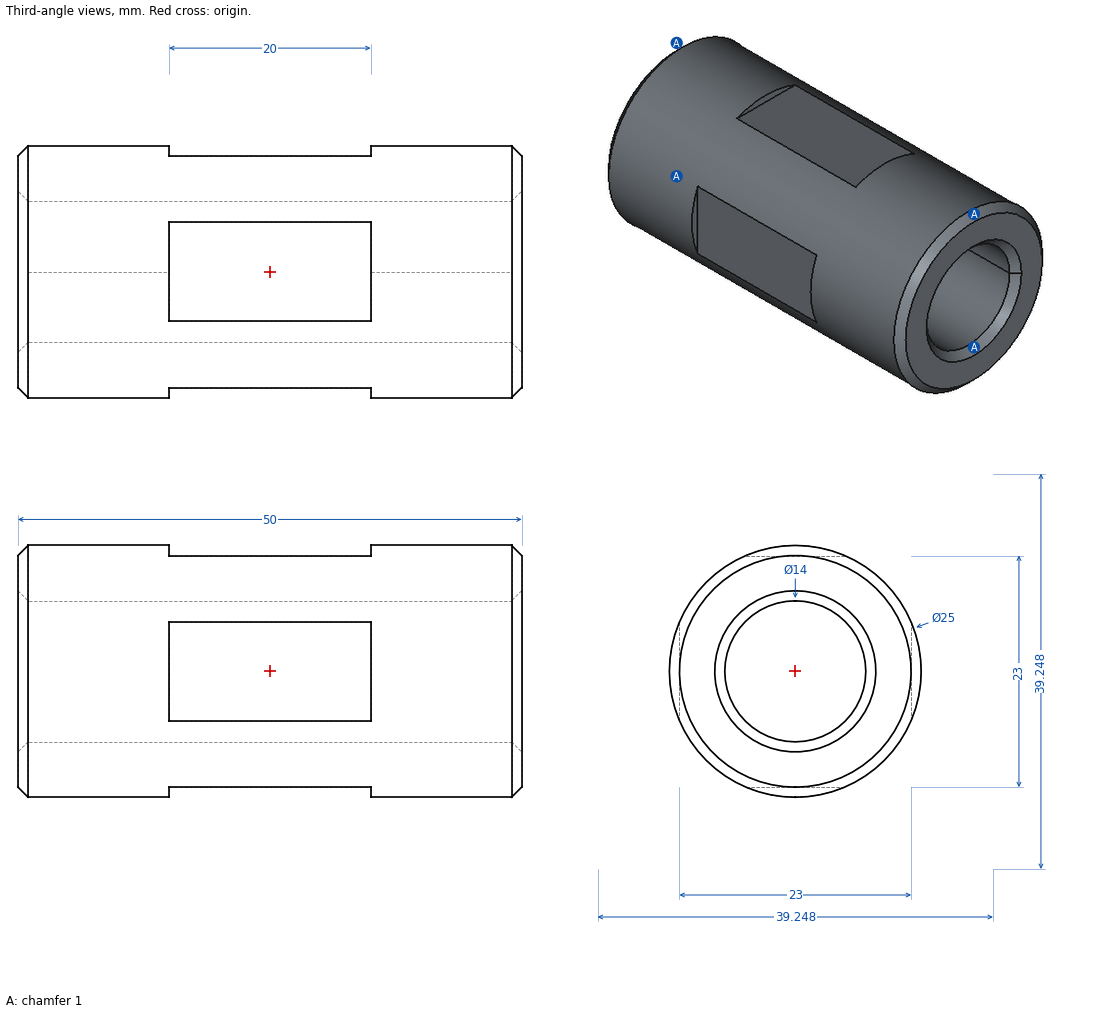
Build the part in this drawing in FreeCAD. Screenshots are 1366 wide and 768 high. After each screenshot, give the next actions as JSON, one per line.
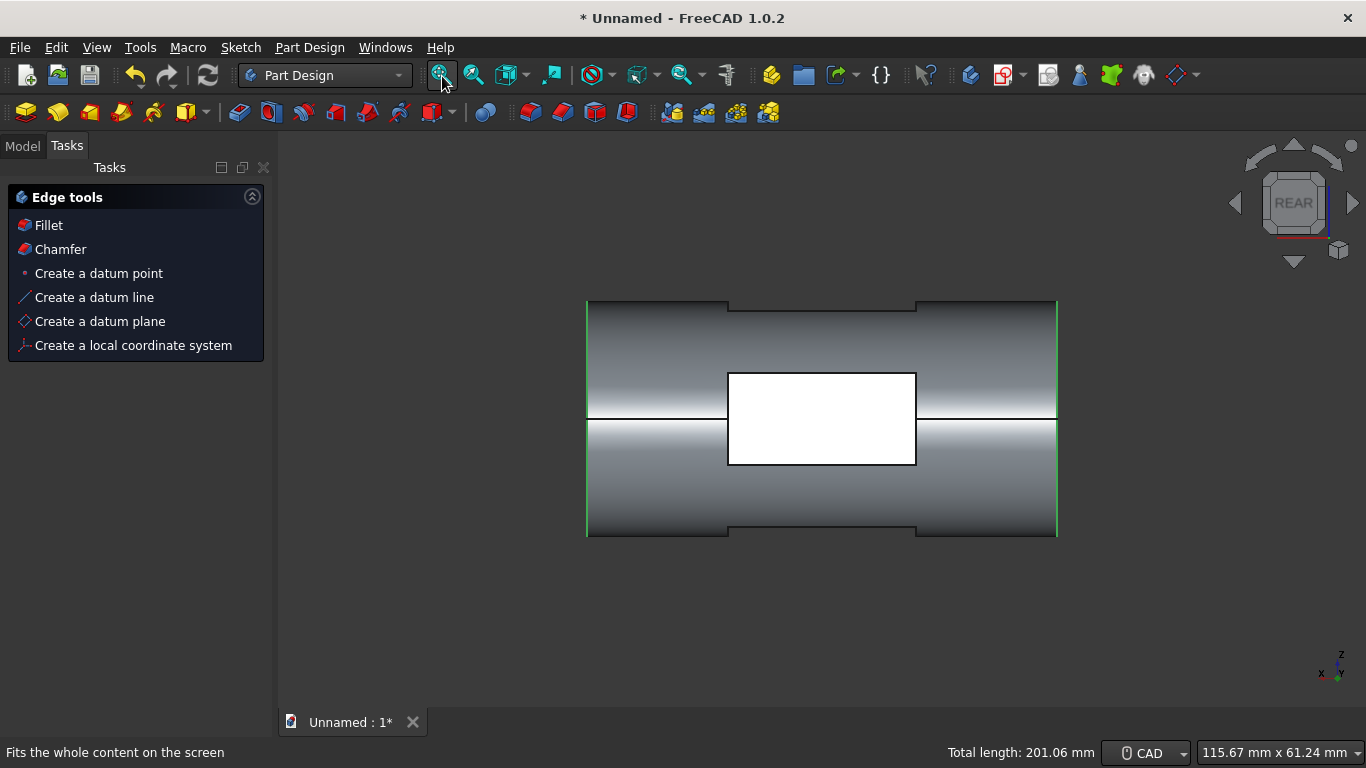
{"action": "key", "text": "6"}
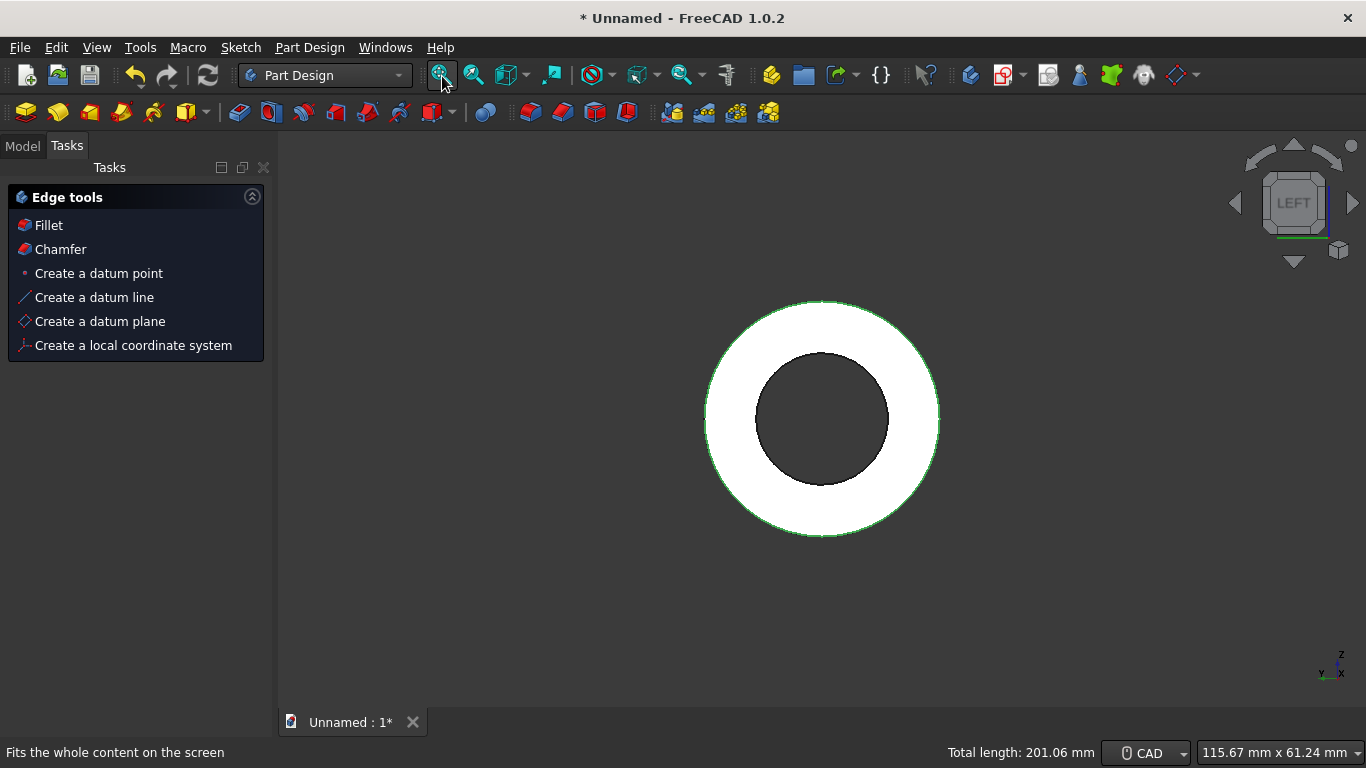
{"action": "key", "text": "v f"}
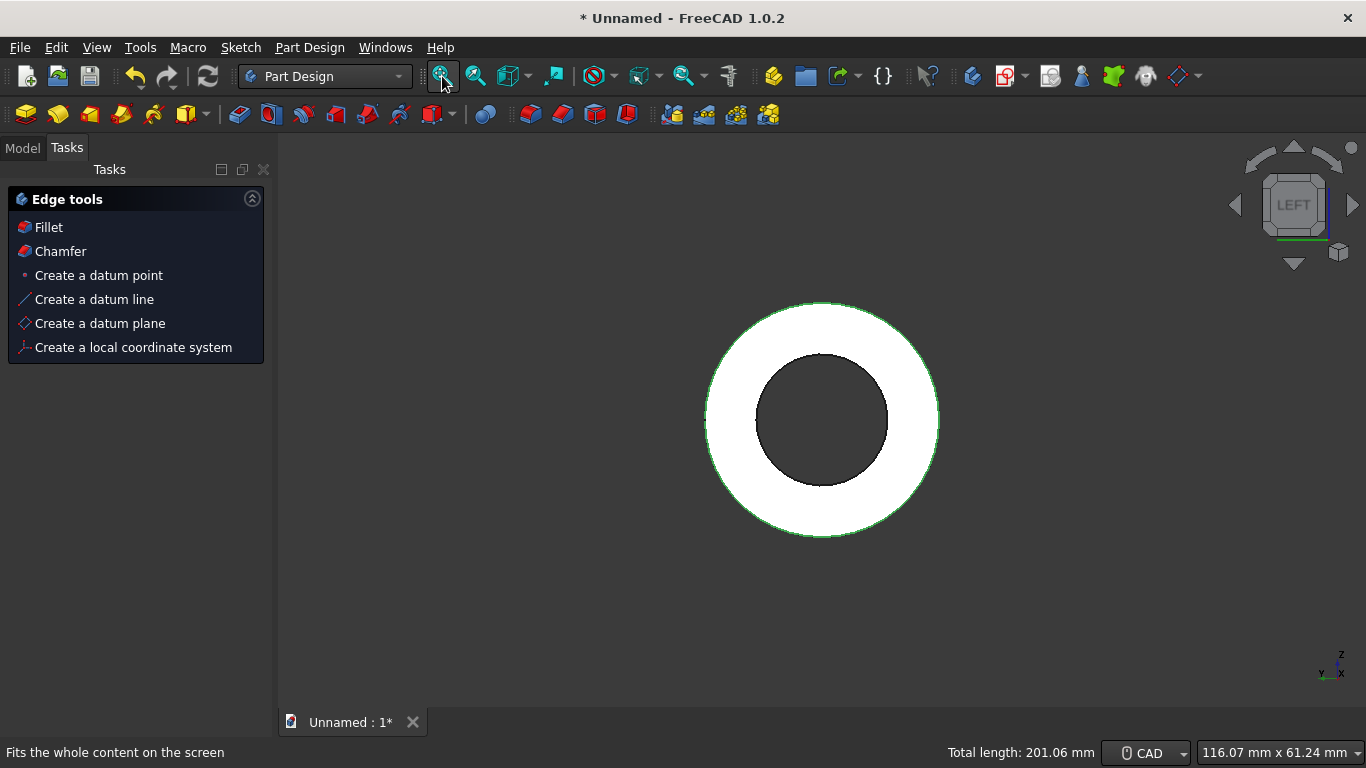
{"action": "left_click", "coordinate": [888, 419], "text": "ctrl"}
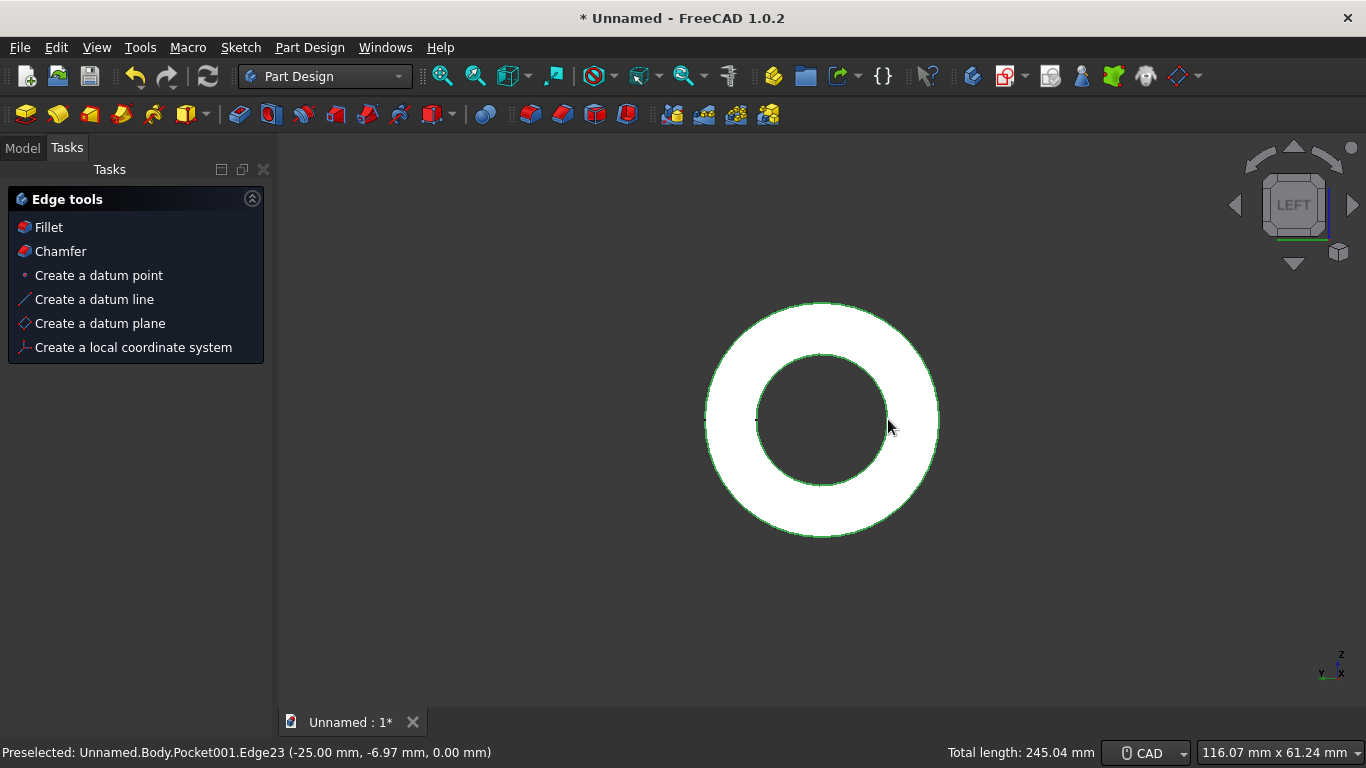
{"action": "left_click", "coordinate": [564, 114]}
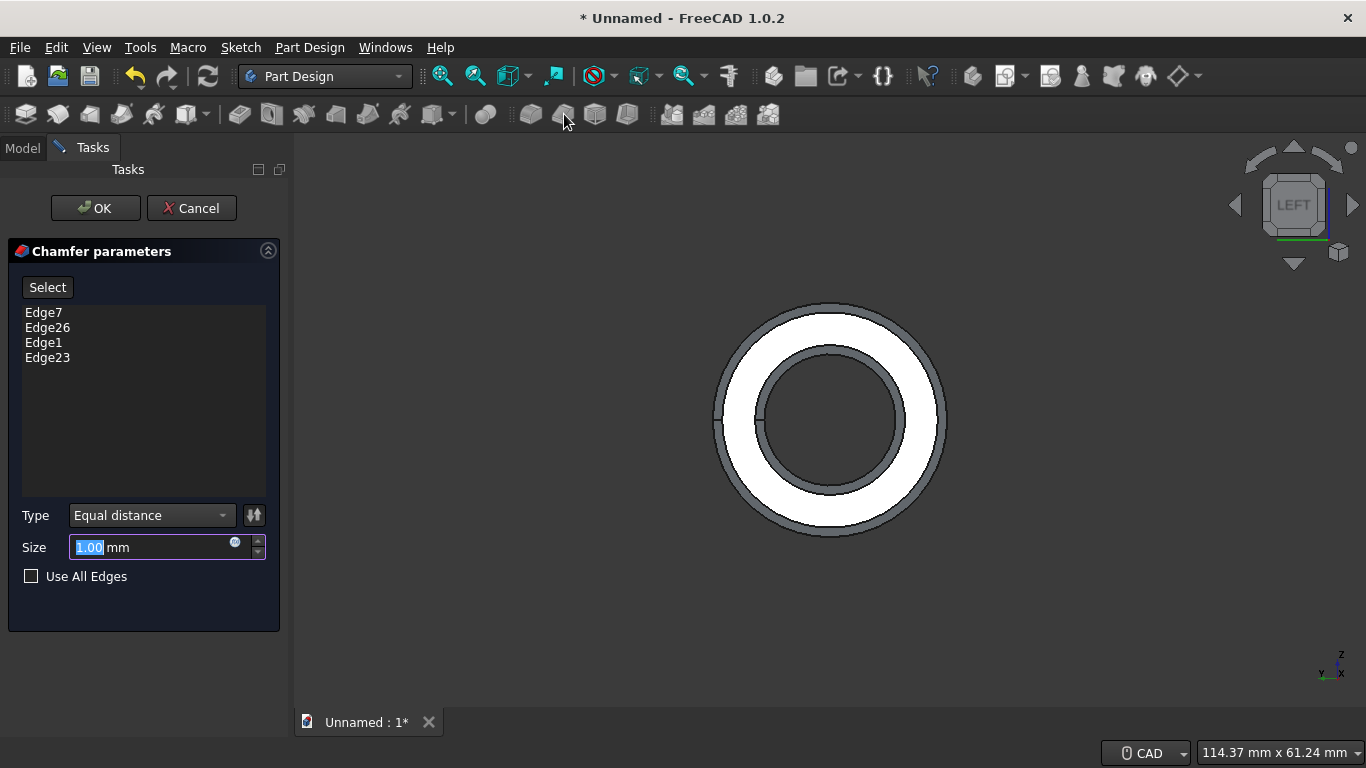
{"action": "type", "text": "1"}
{"action": "key", "text": "Tab"}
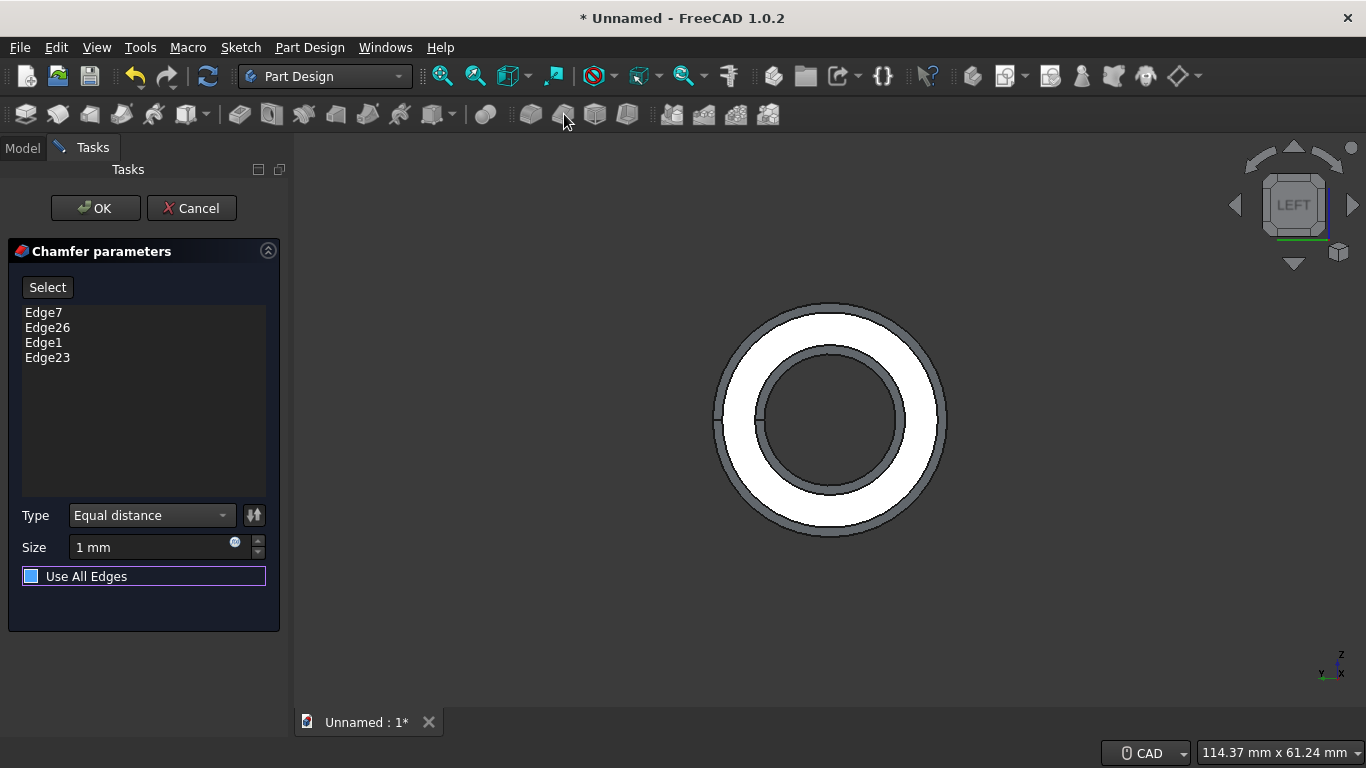
{"action": "left_click", "coordinate": [96, 208]}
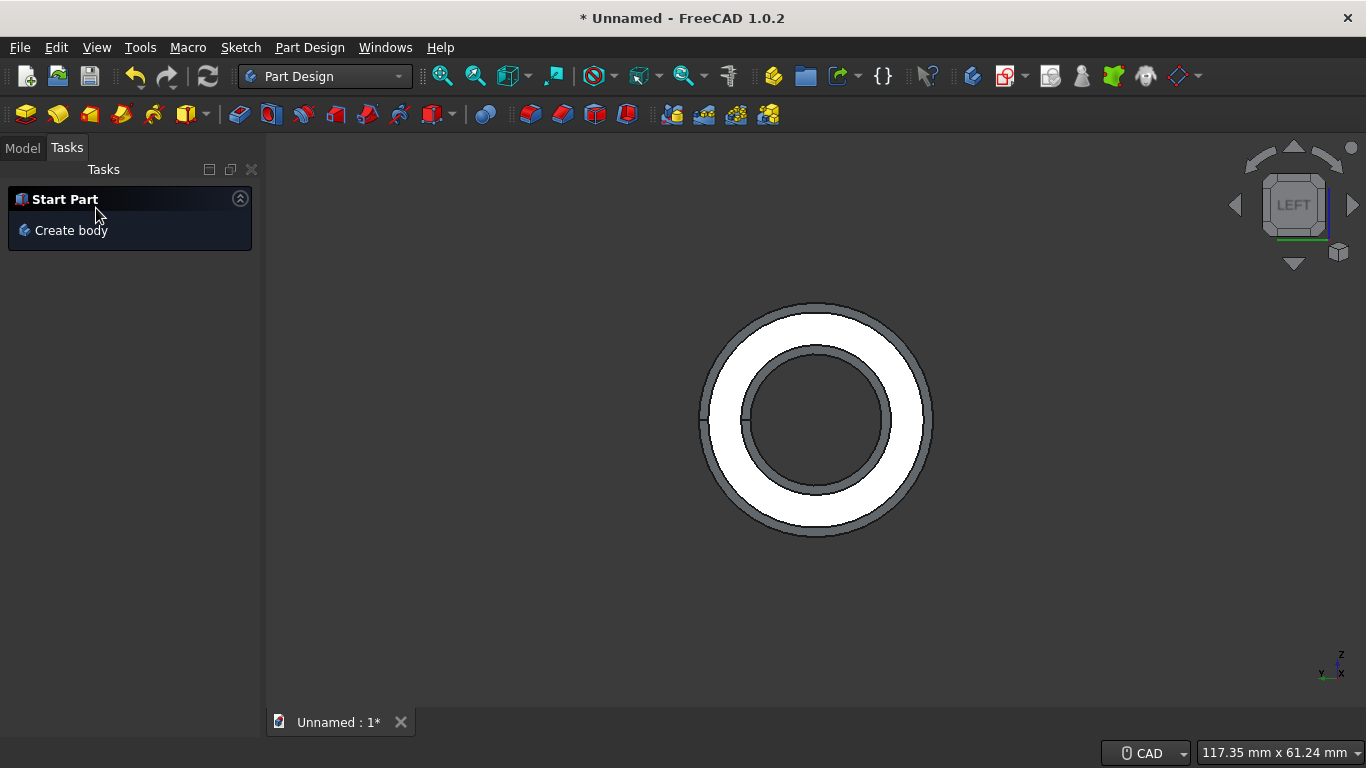
{"action": "key", "text": "0"}